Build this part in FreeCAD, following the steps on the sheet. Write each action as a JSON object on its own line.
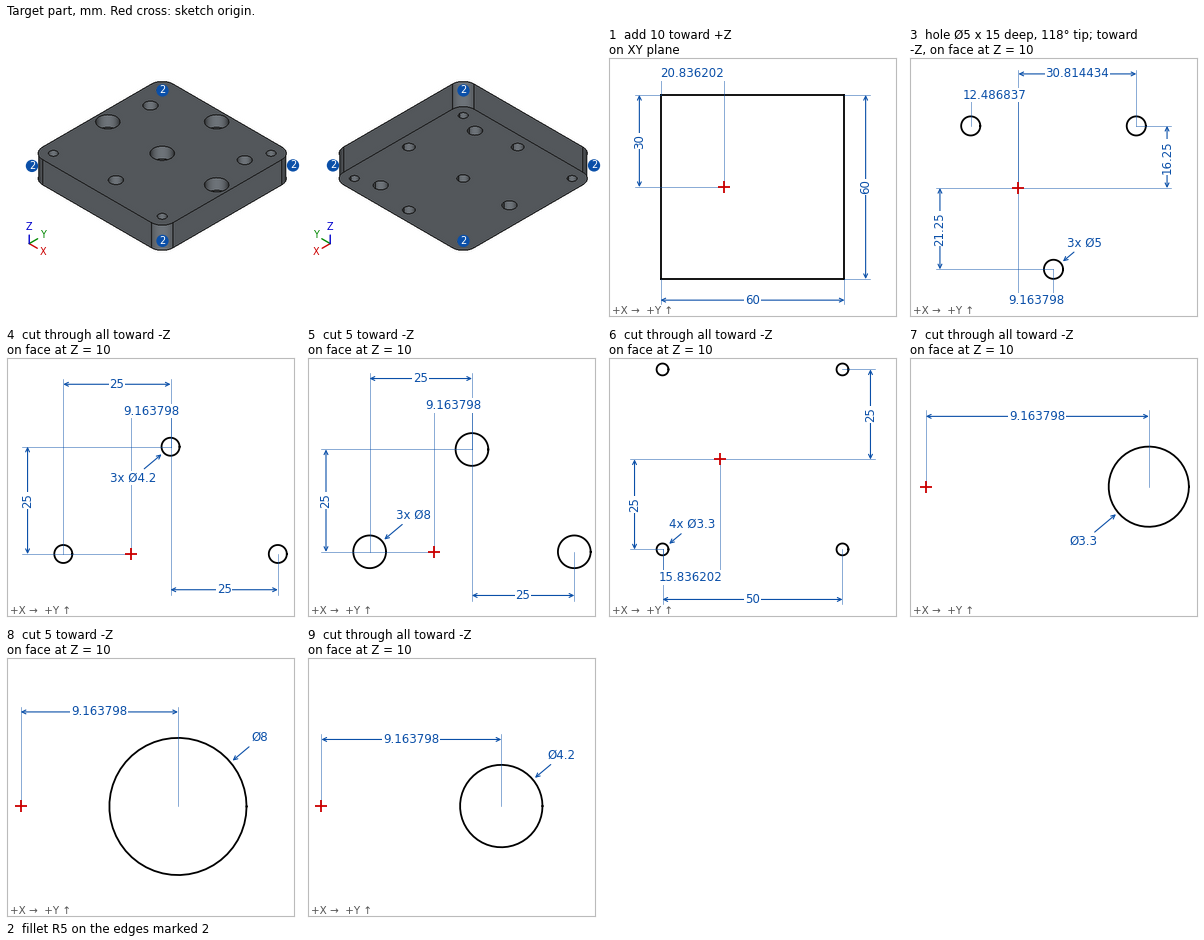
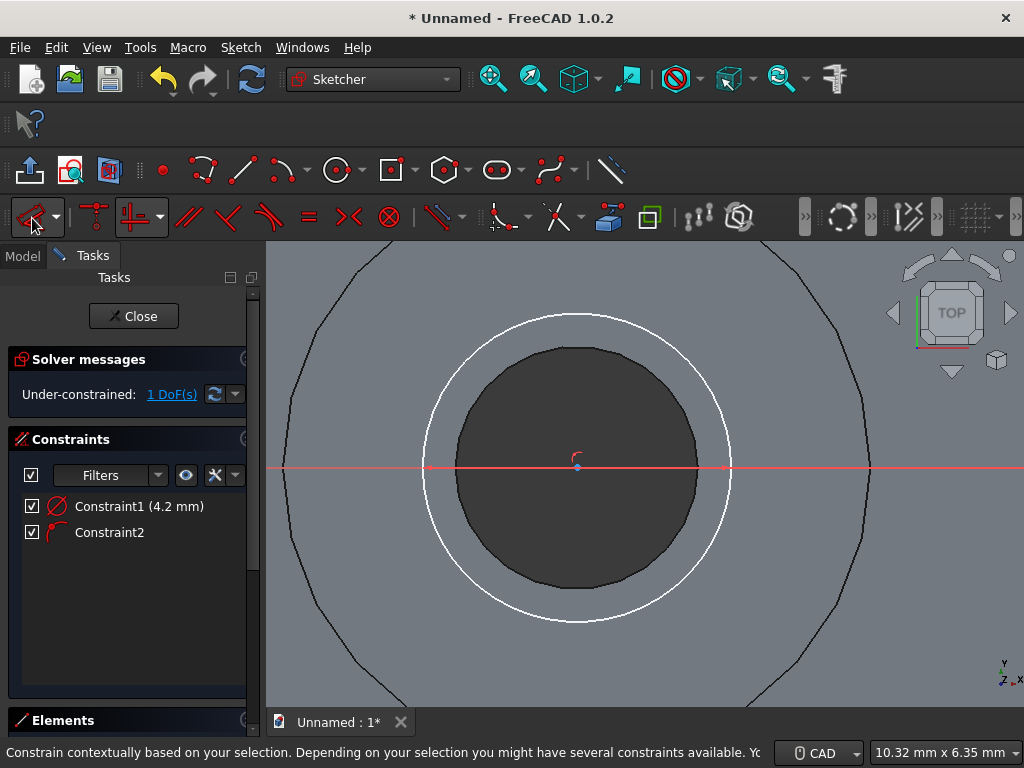
{"action": "left_click", "coordinate": [577, 468]}
{"action": "left_click", "coordinate": [370, 502]}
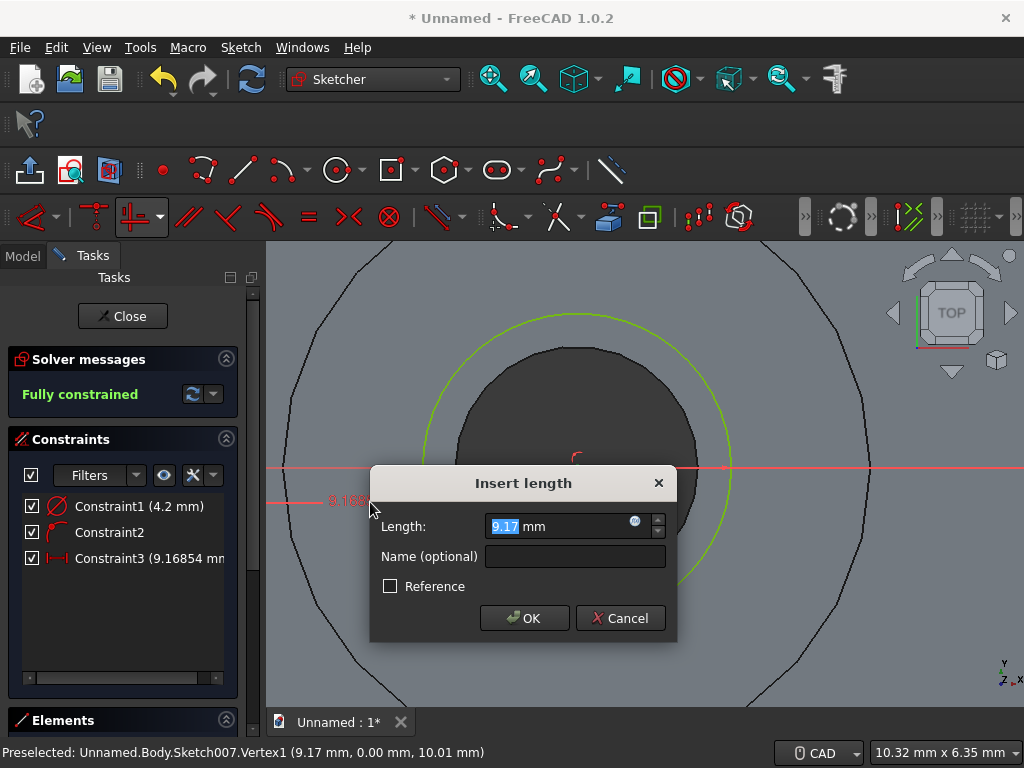
{"action": "type", "text": "9.163798"}
{"action": "key", "text": "Return"}
{"action": "key", "text": "Escape"}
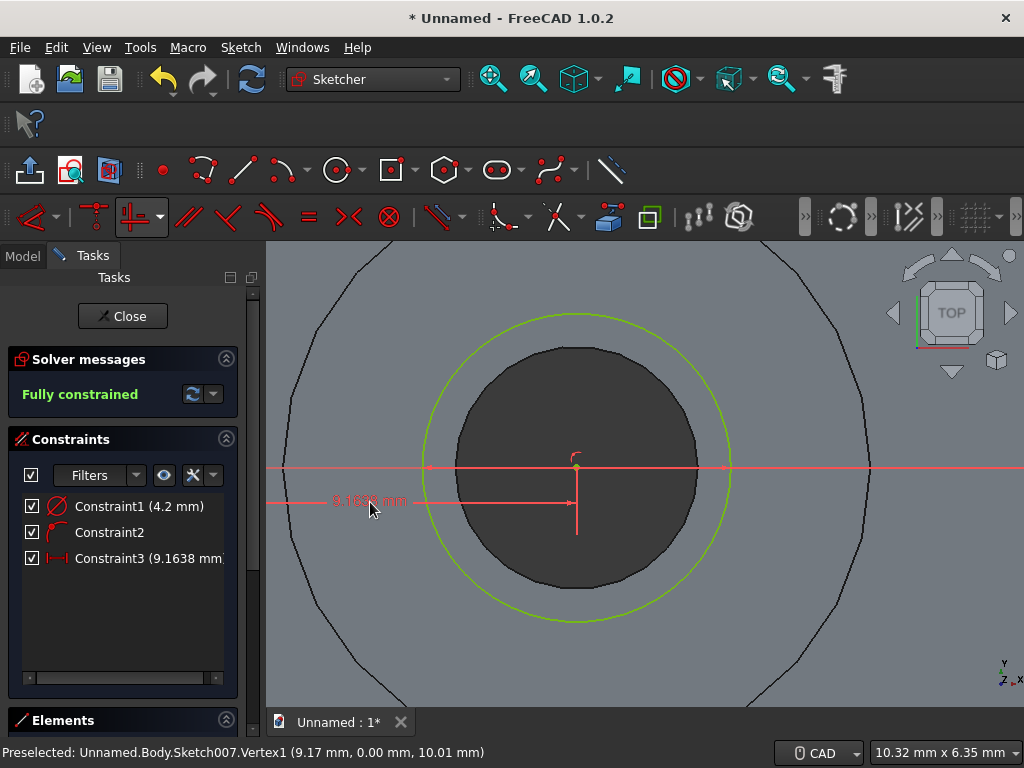
{"action": "left_click", "coordinate": [123, 316]}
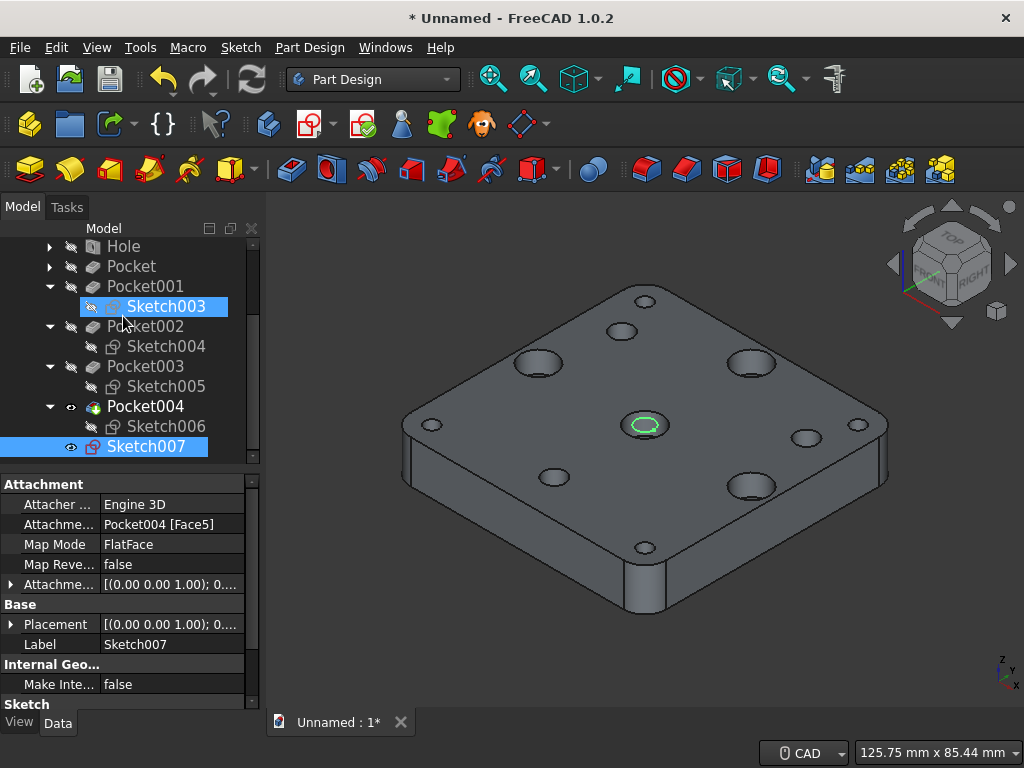
{"action": "left_click", "coordinate": [292, 170]}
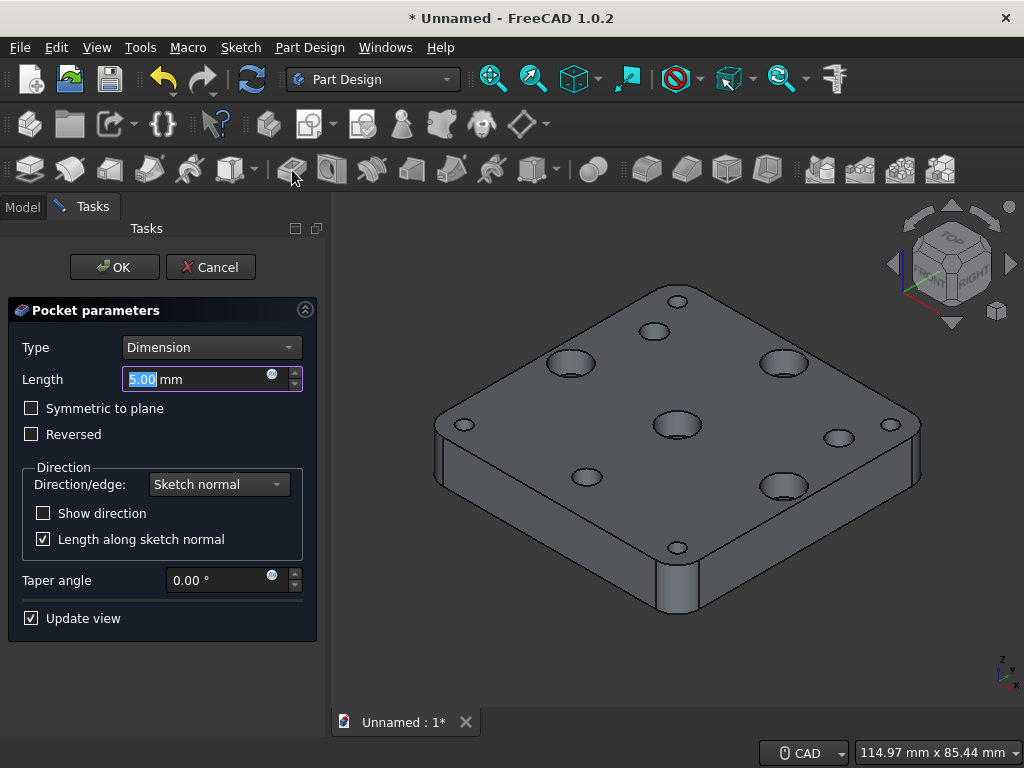
{"action": "left_click", "coordinate": [212, 348]}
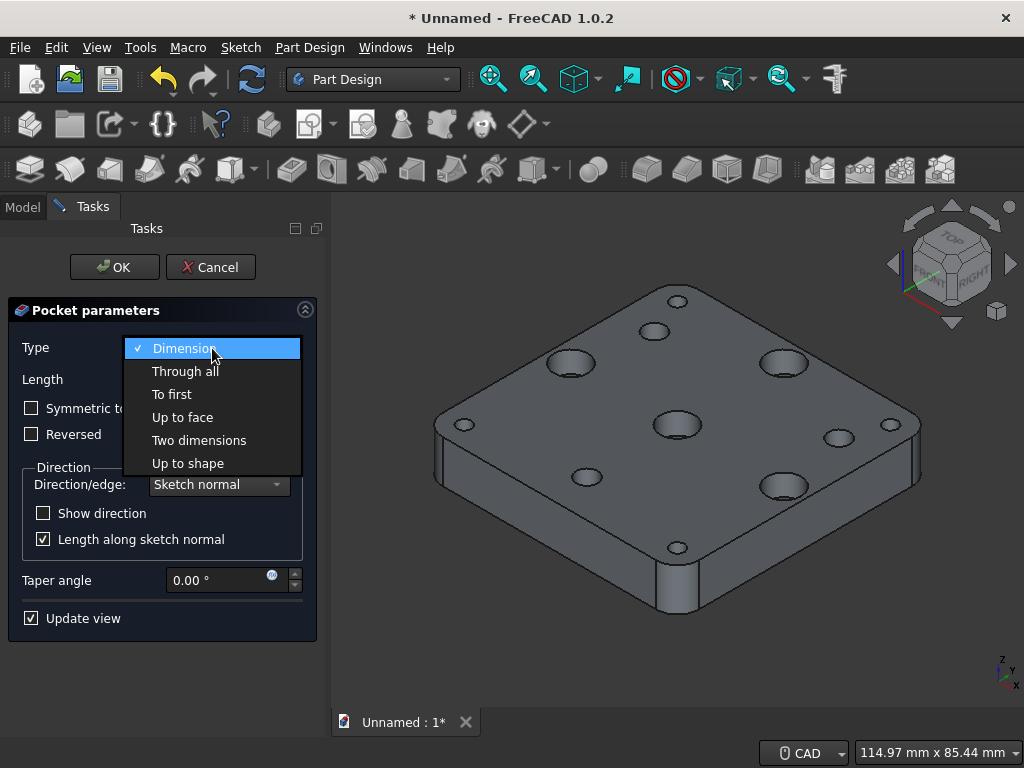
{"action": "left_click", "coordinate": [212, 372]}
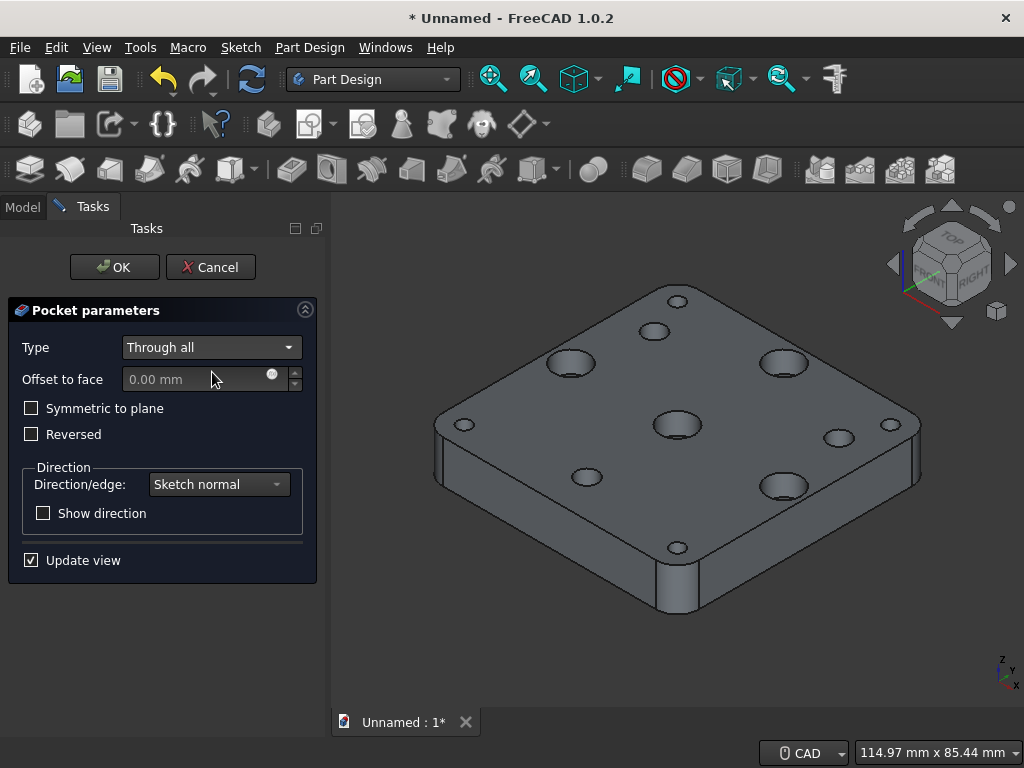
{"action": "left_click", "coordinate": [115, 267]}